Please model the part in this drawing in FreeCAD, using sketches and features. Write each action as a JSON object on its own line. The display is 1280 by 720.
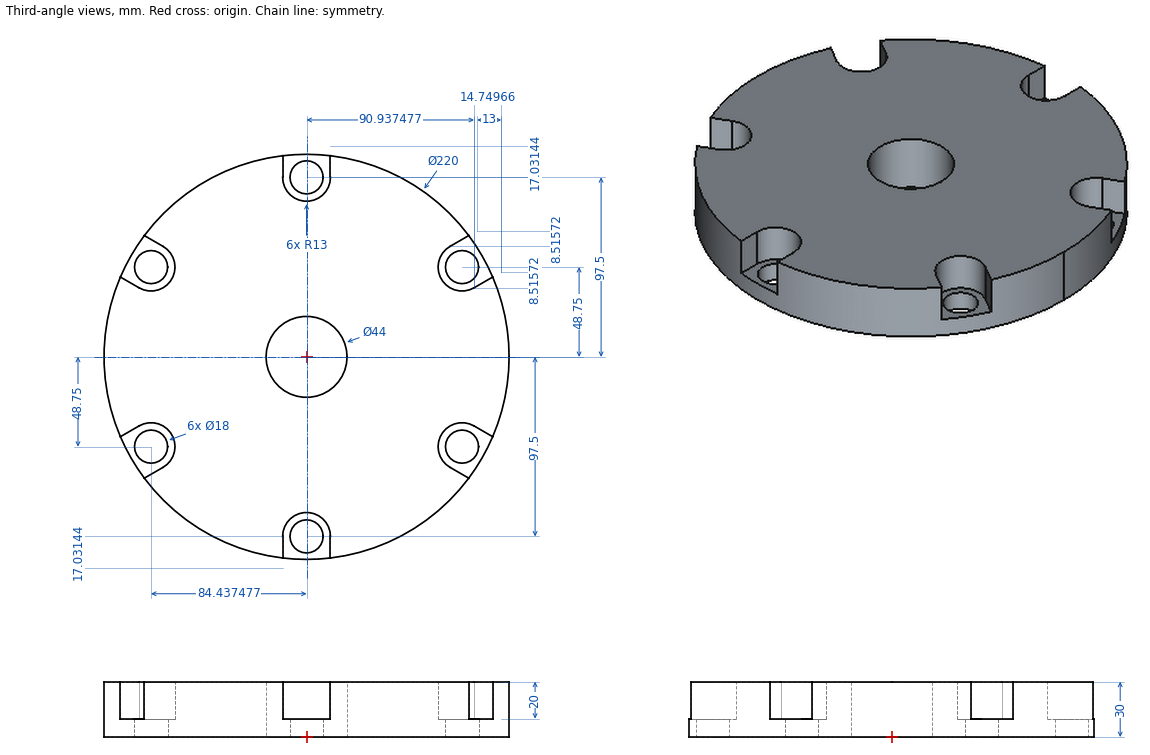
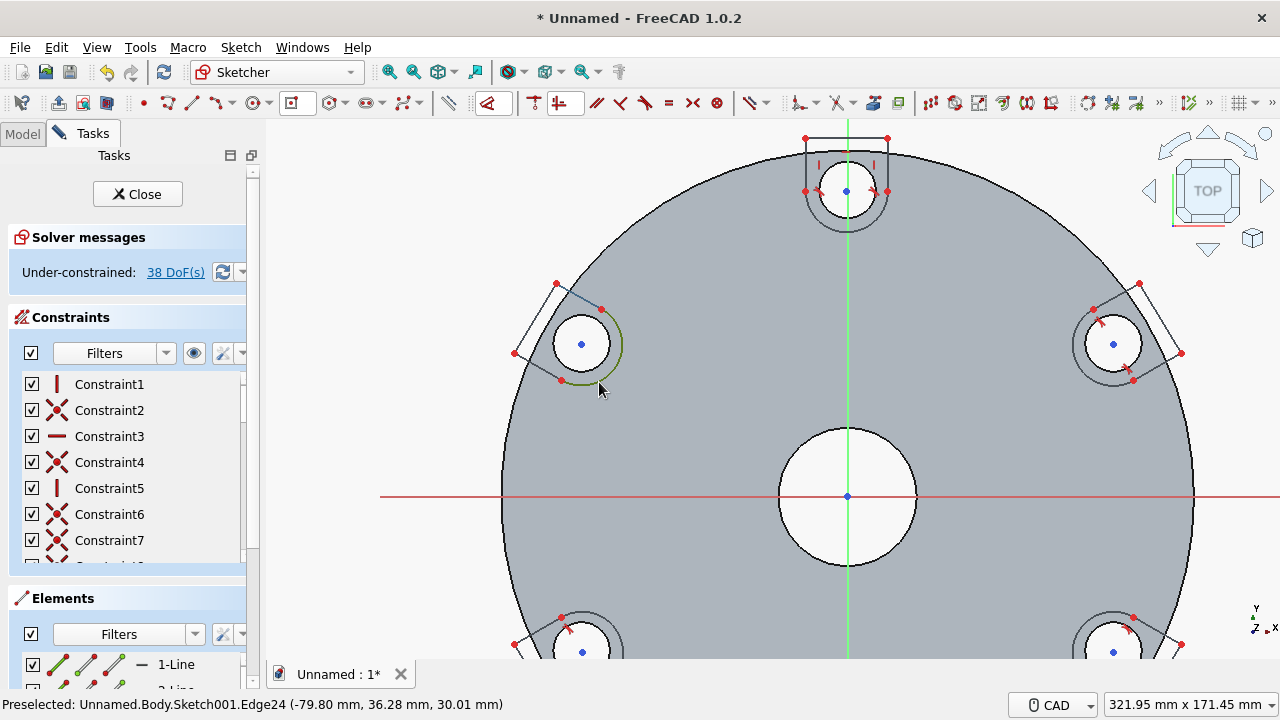
{"action": "left_click", "coordinate": [646, 104]}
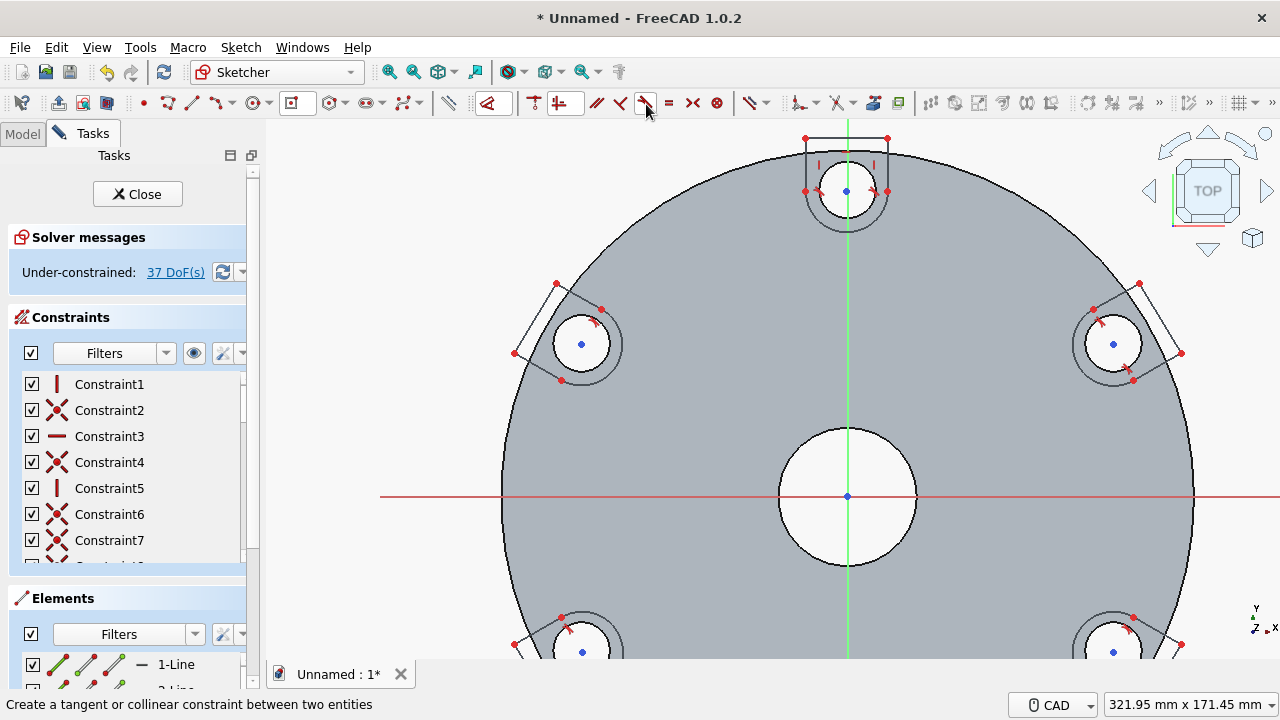
{"action": "left_click", "coordinate": [529, 361]}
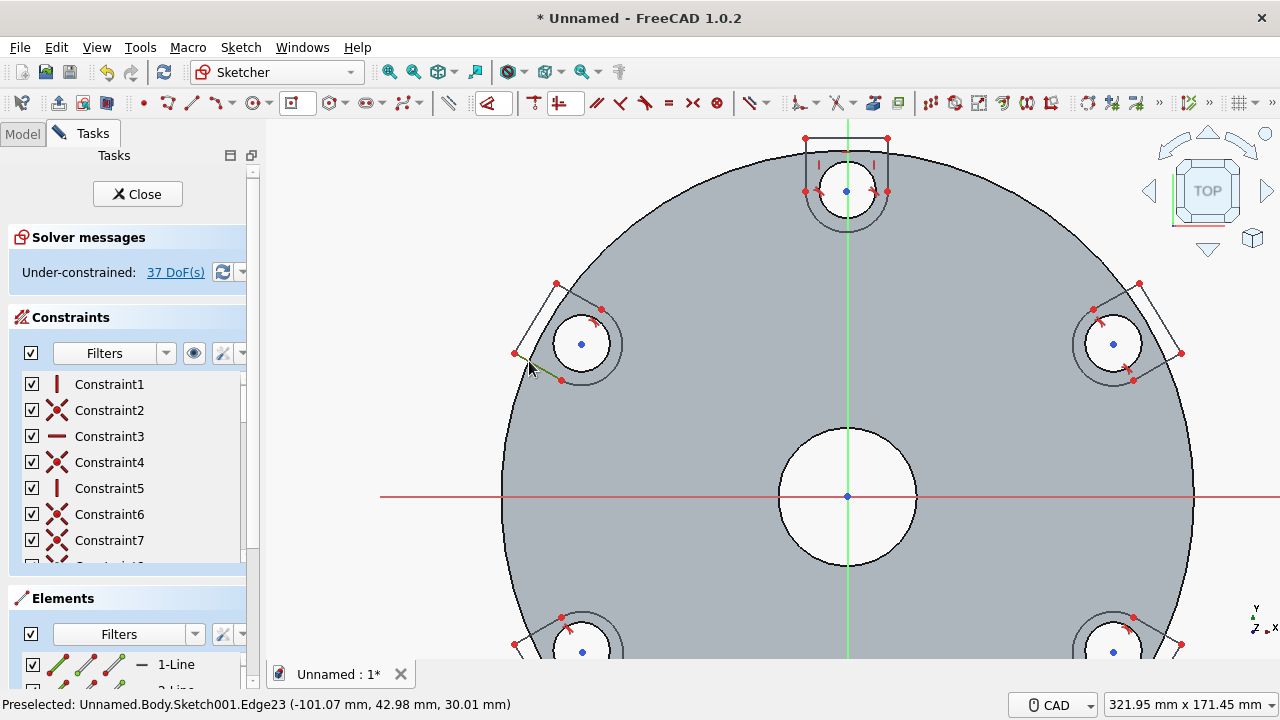
{"action": "left_click", "coordinate": [599, 382]}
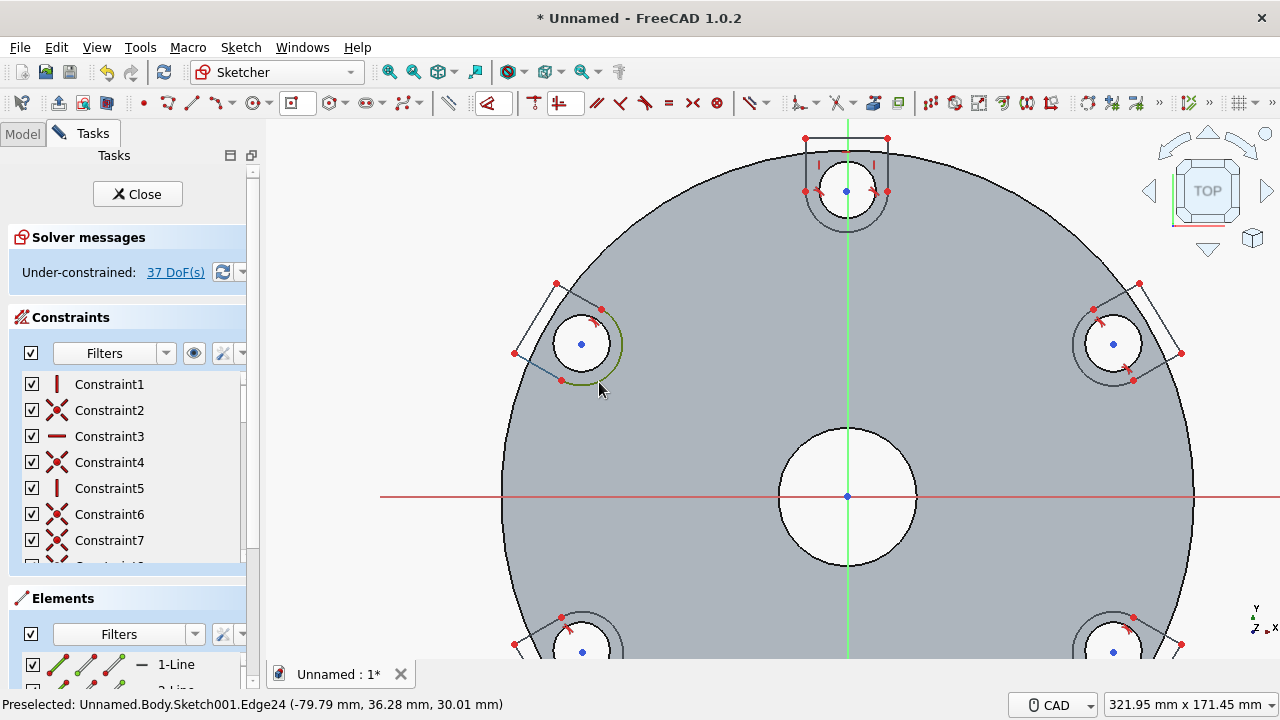
{"action": "left_click", "coordinate": [646, 104]}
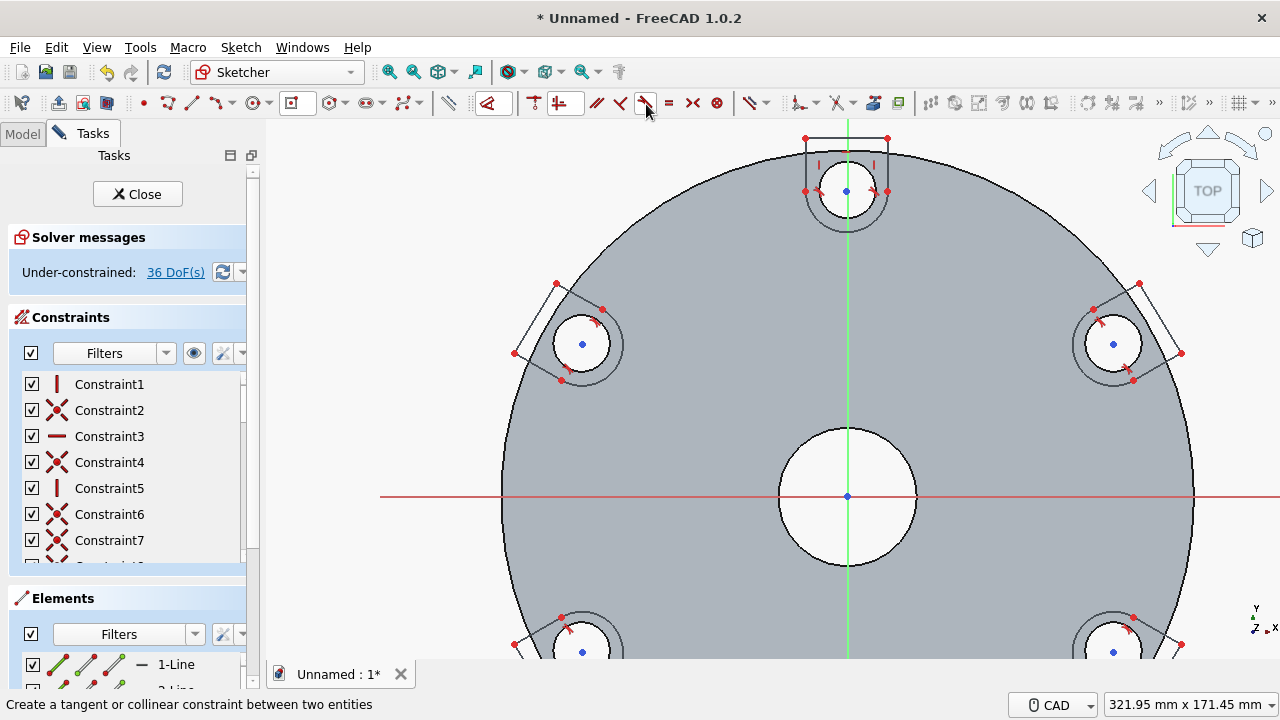
{"action": "left_click", "coordinate": [823, 224]}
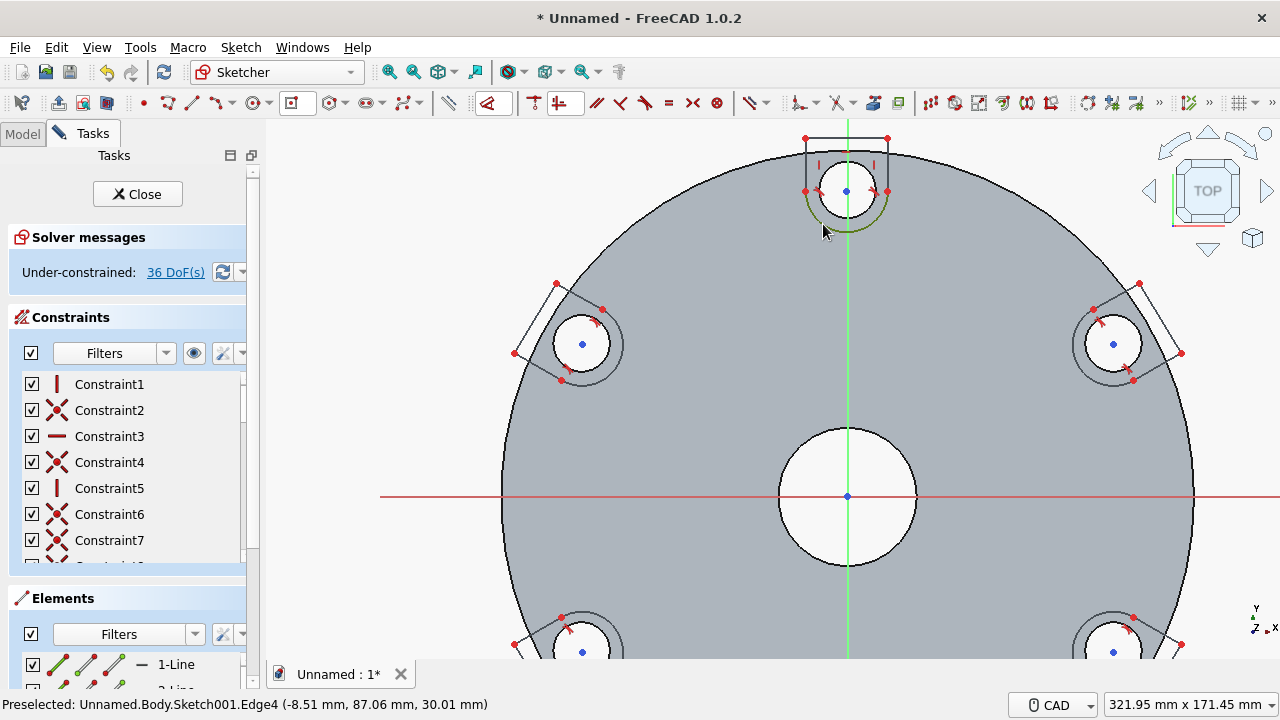
{"action": "left_click", "coordinate": [1073, 340]}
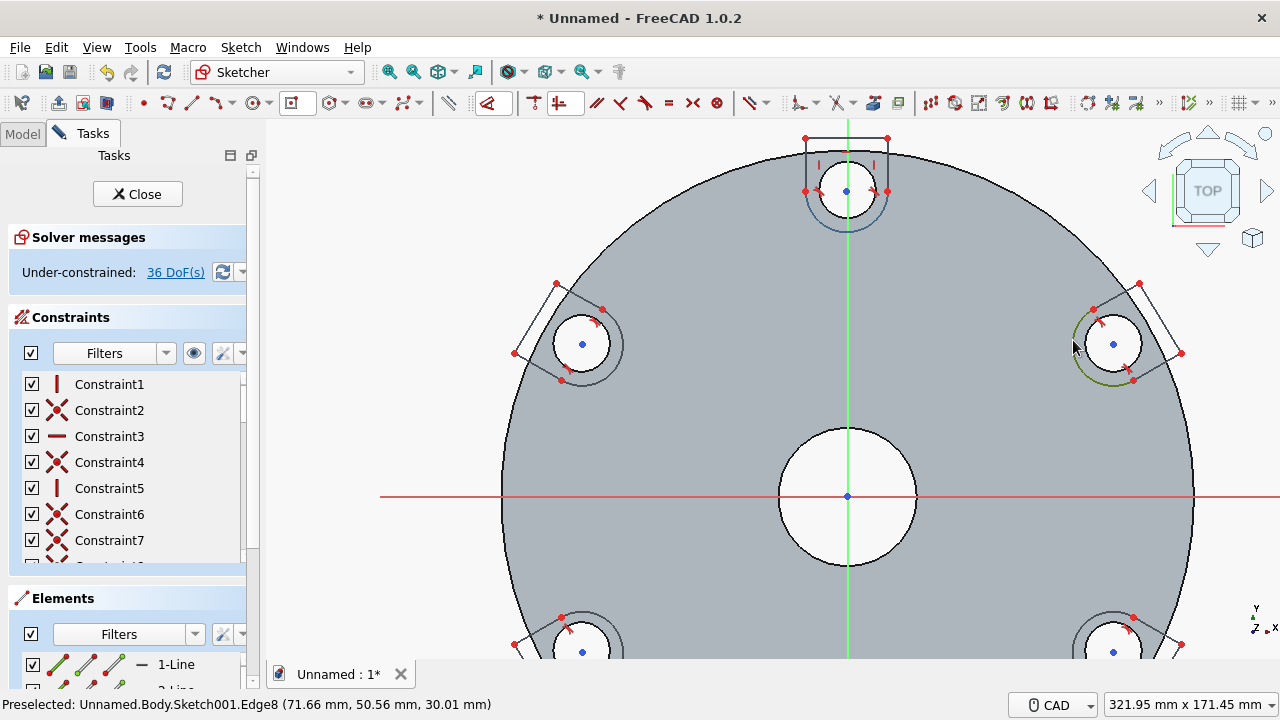
{"action": "left_click", "coordinate": [1097, 615]}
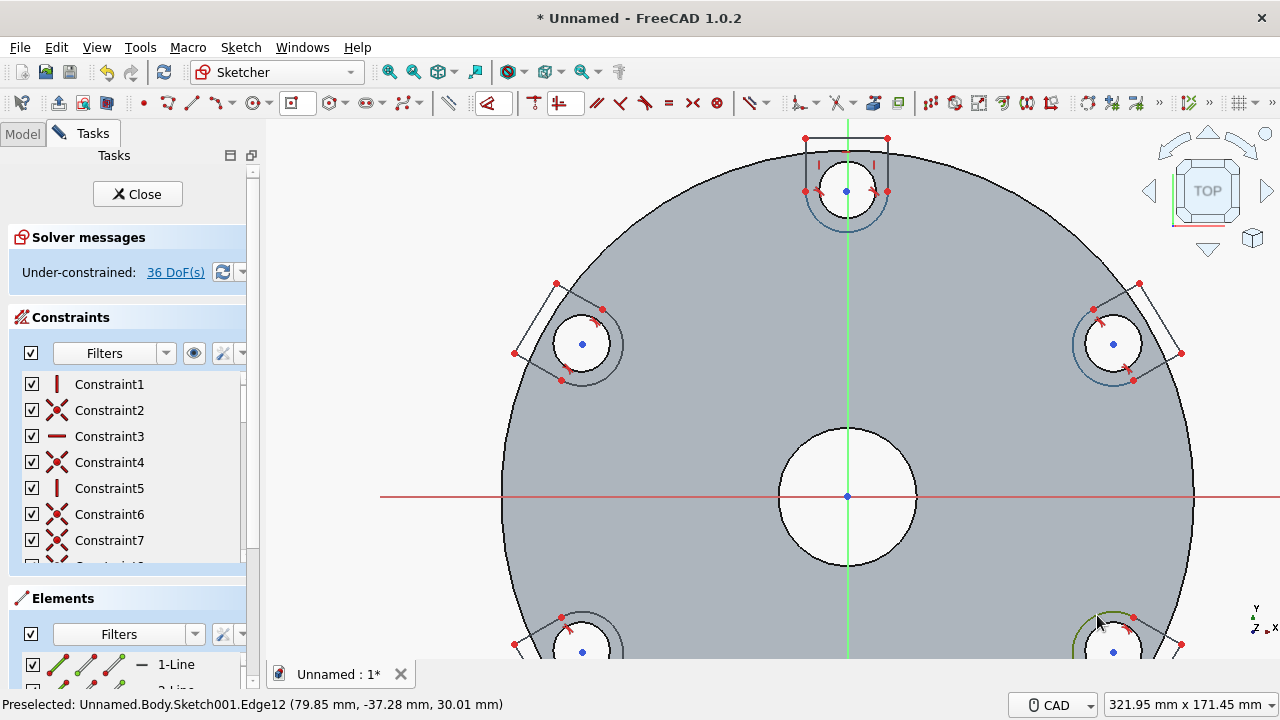
{"action": "scroll", "coordinate": [588, 301], "scroll_direction": "down", "scroll_amount": 4}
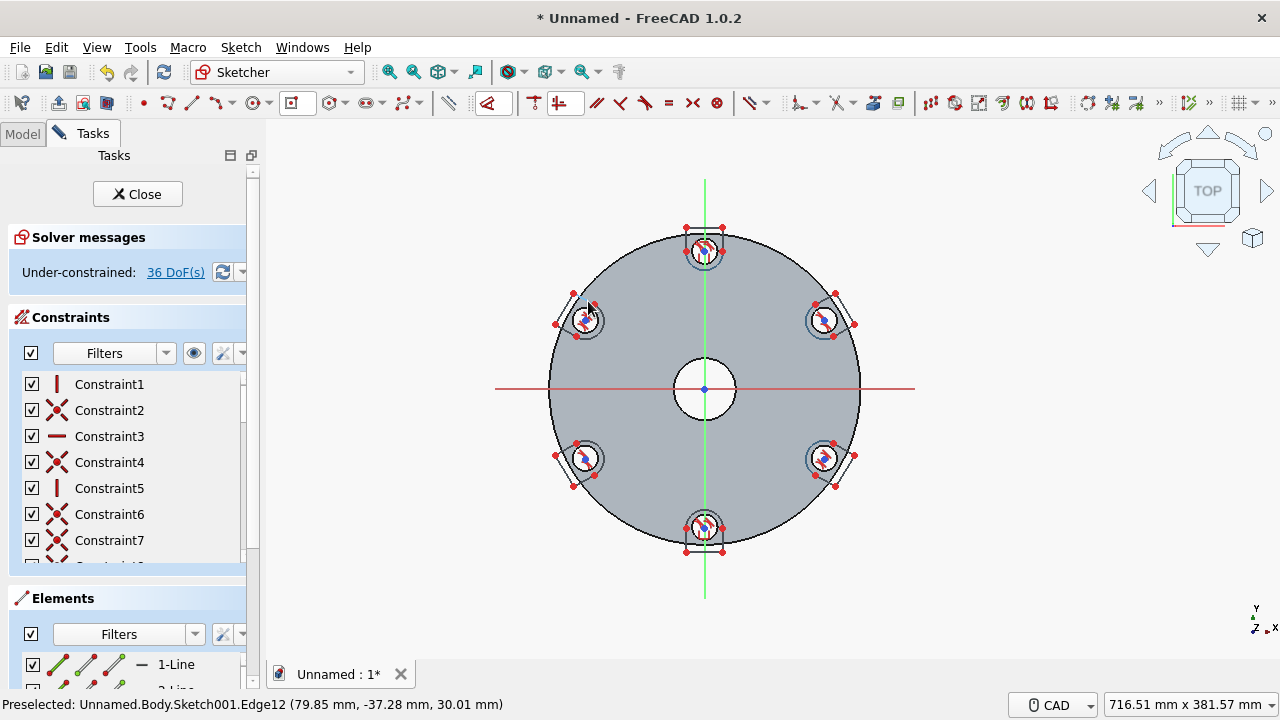
{"action": "scroll", "coordinate": [715, 513], "scroll_direction": "up", "scroll_amount": 2}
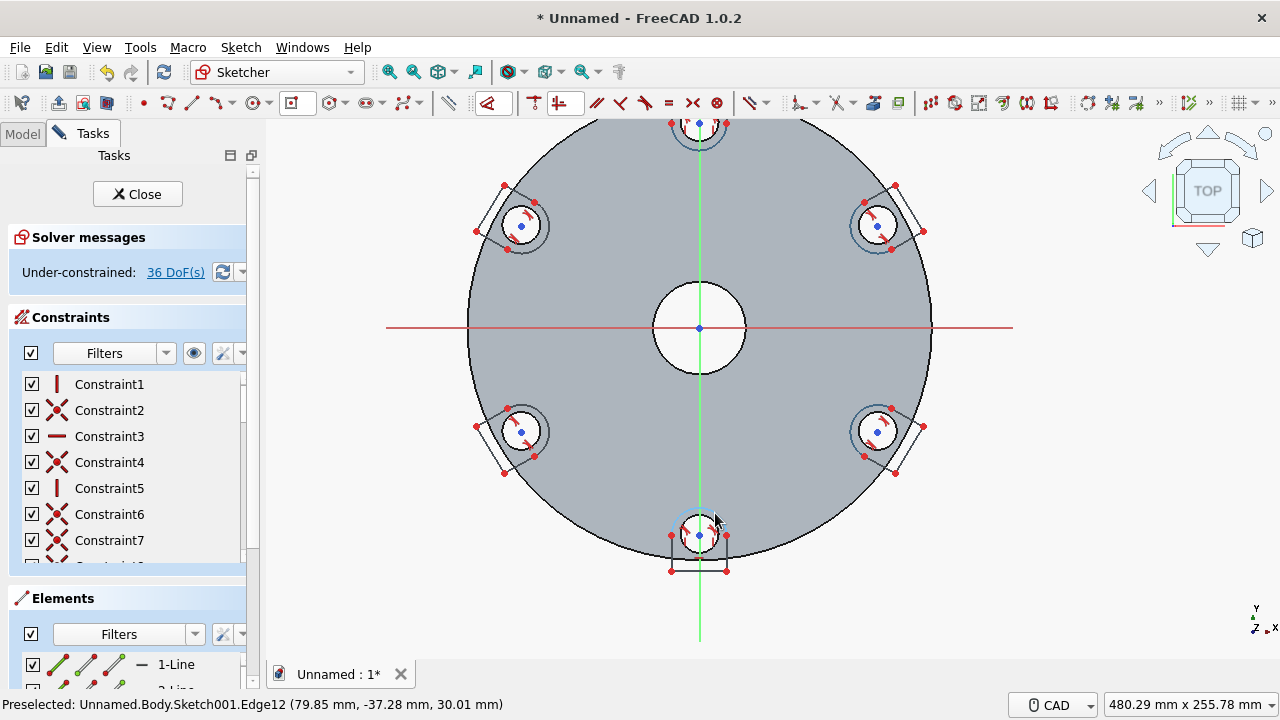
{"action": "left_click", "coordinate": [715, 513]}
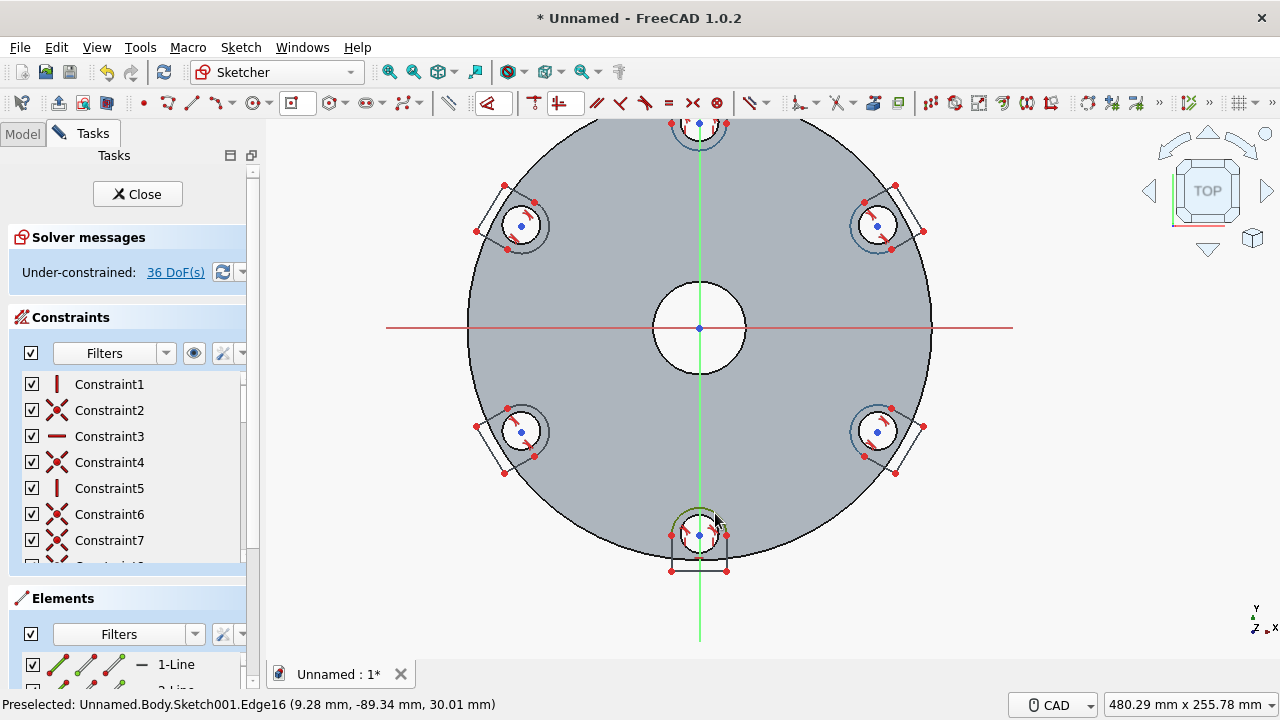
{"action": "left_click", "coordinate": [549, 436]}